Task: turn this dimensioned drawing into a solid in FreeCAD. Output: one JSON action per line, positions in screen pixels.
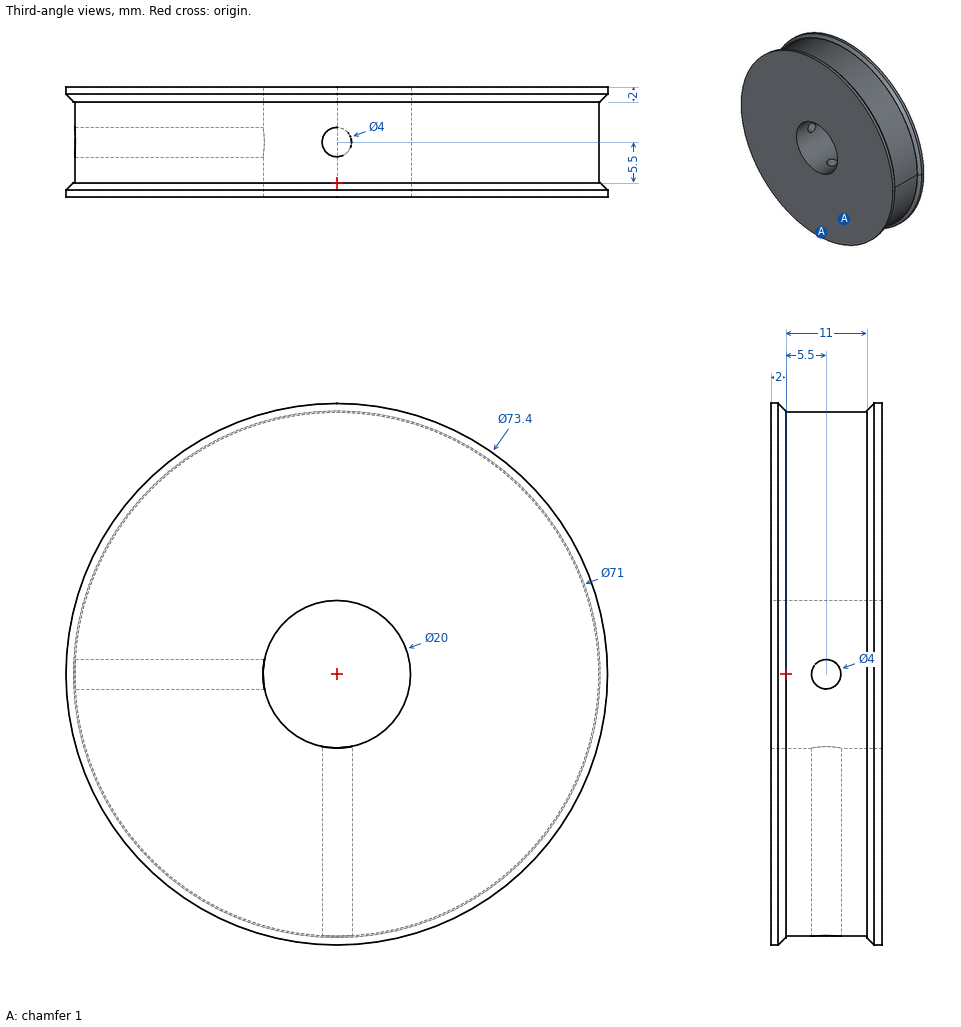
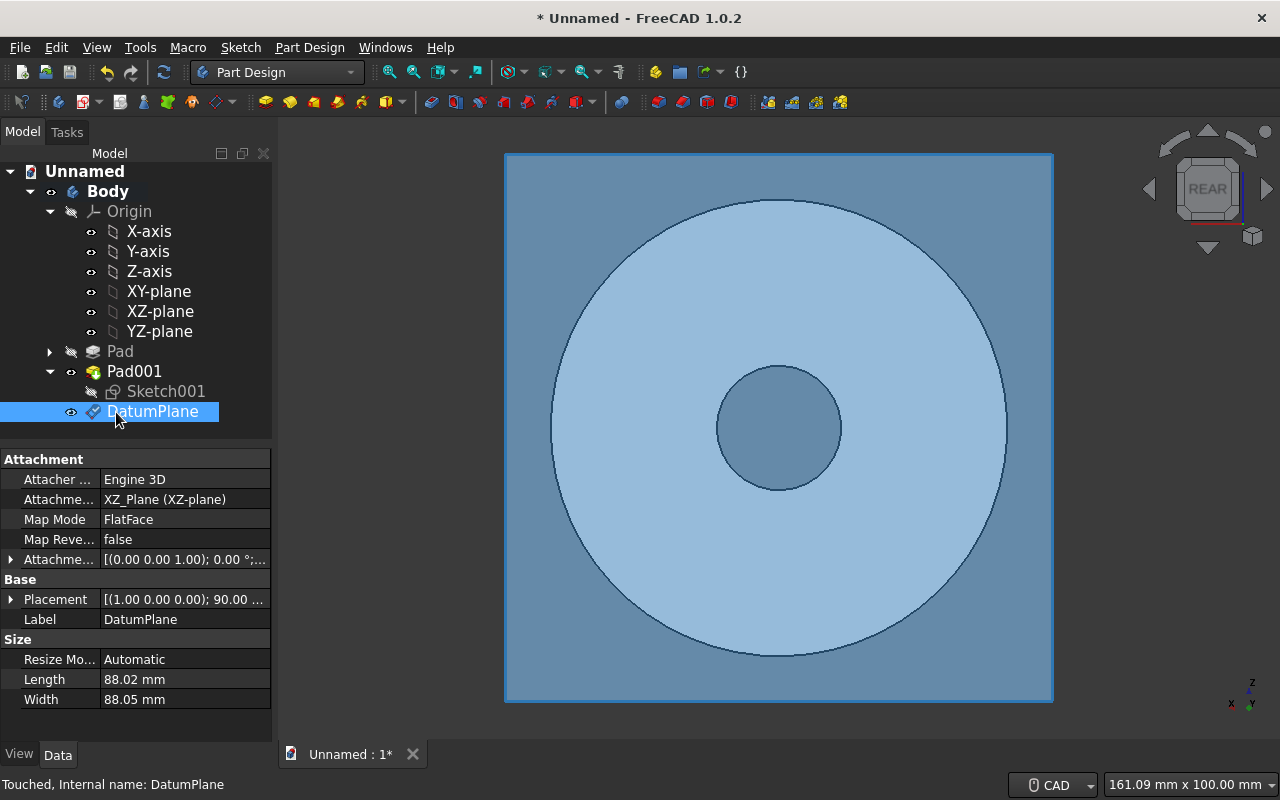
{"action": "left_click", "coordinate": [84, 102]}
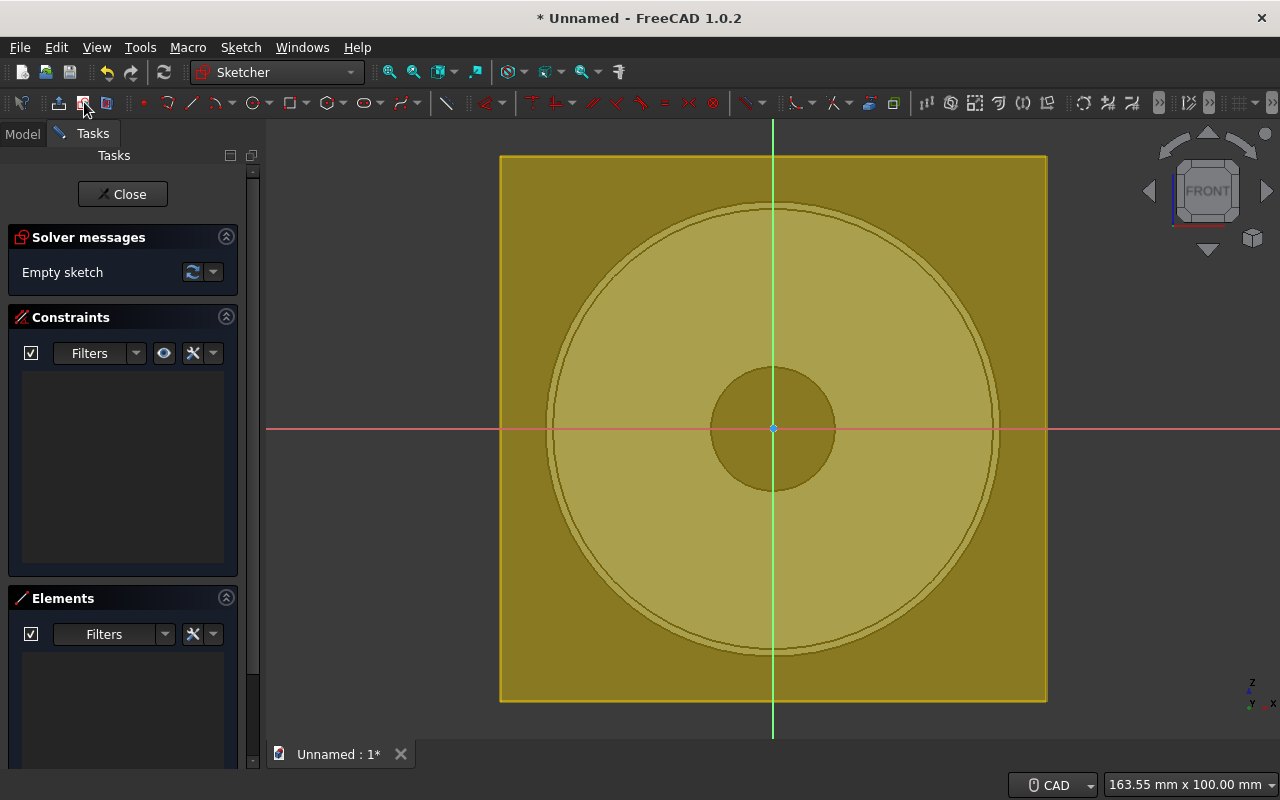
{"action": "left_click", "coordinate": [254, 104]}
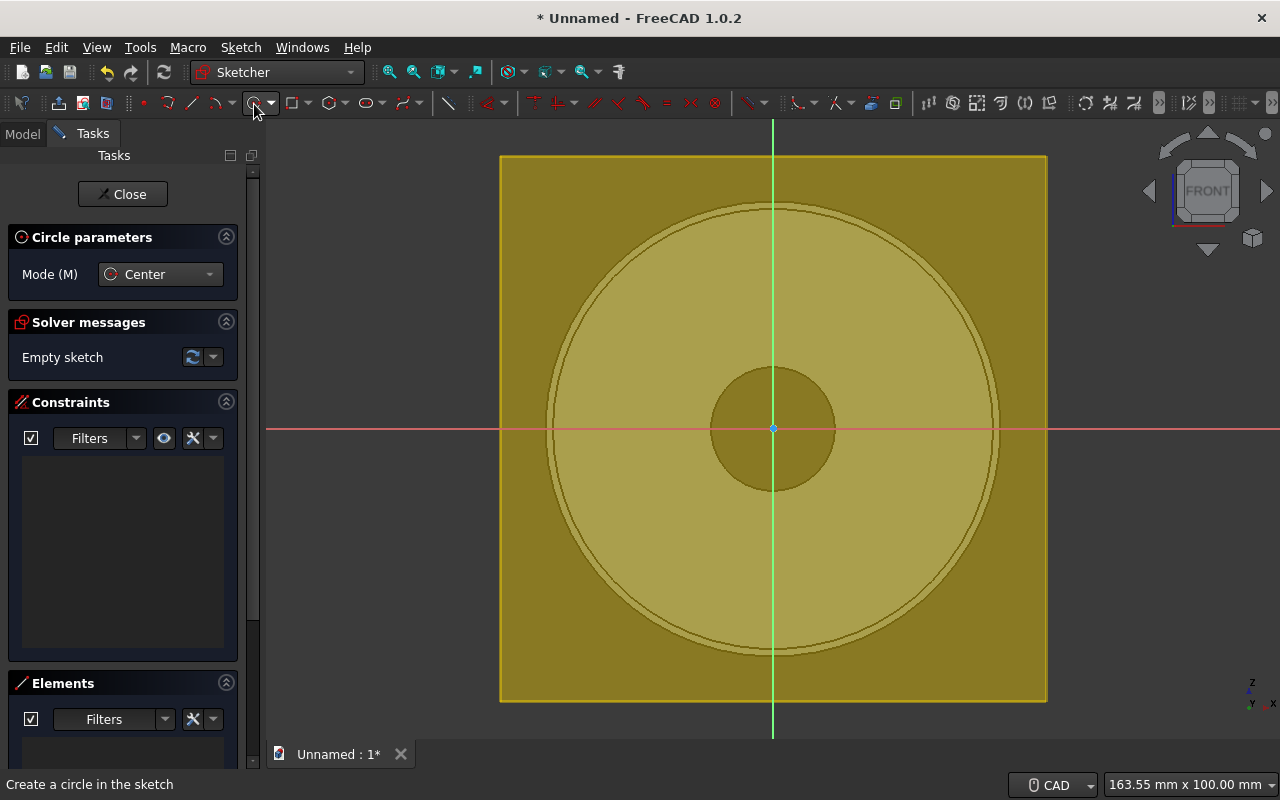
{"action": "left_click", "coordinate": [773, 429]}
{"action": "left_click", "coordinate": [934, 268]}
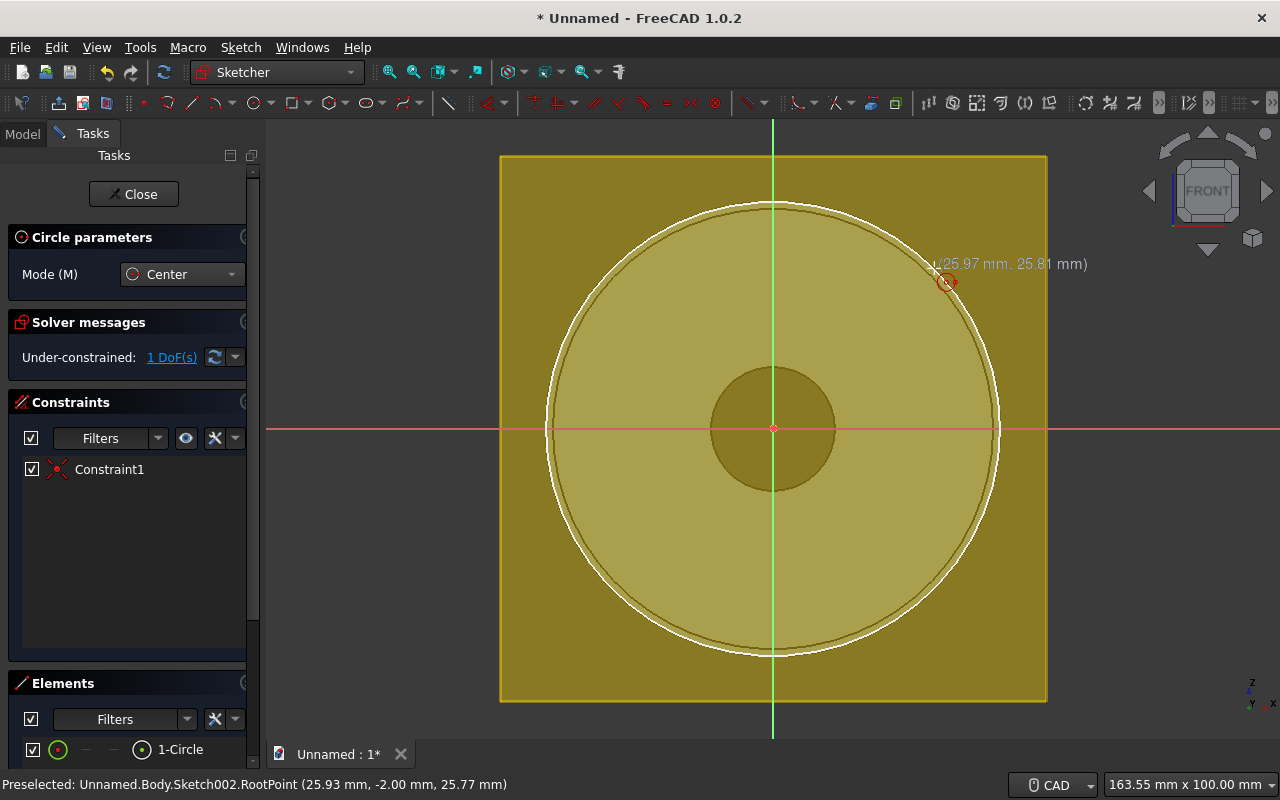
{"action": "left_click", "coordinate": [773, 429]}
{"action": "left_click", "coordinate": [817, 385]}
{"action": "key", "text": "Escape"}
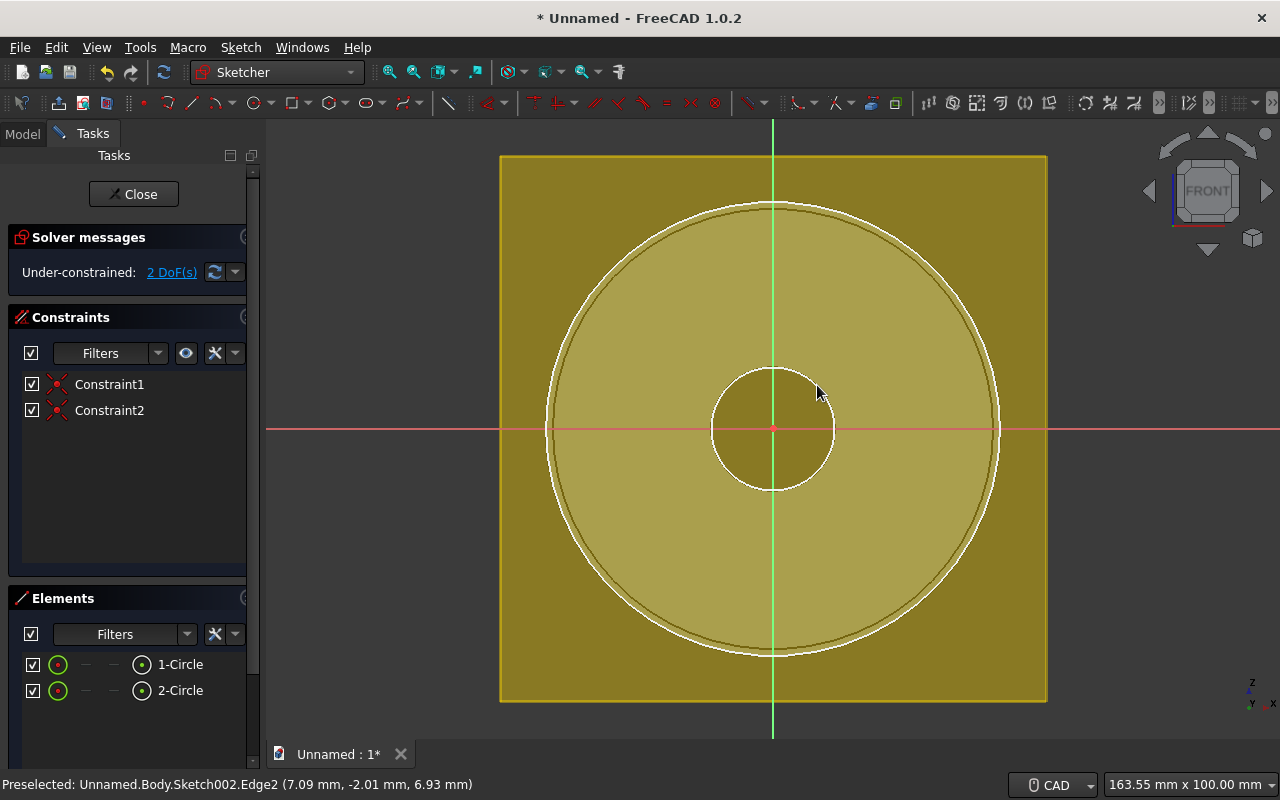
{"action": "left_click", "coordinate": [488, 104]}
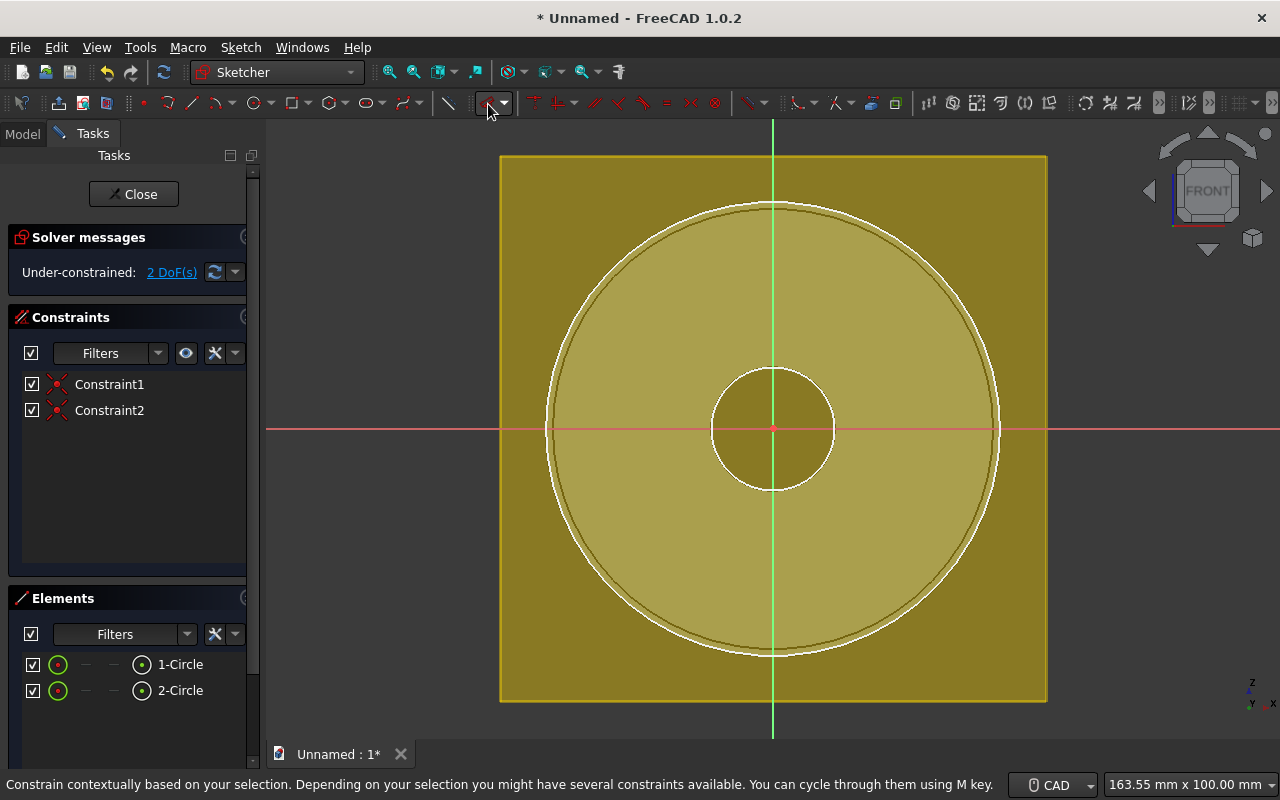
{"action": "left_click", "coordinate": [933, 268]}
{"action": "left_click", "coordinate": [956, 245]}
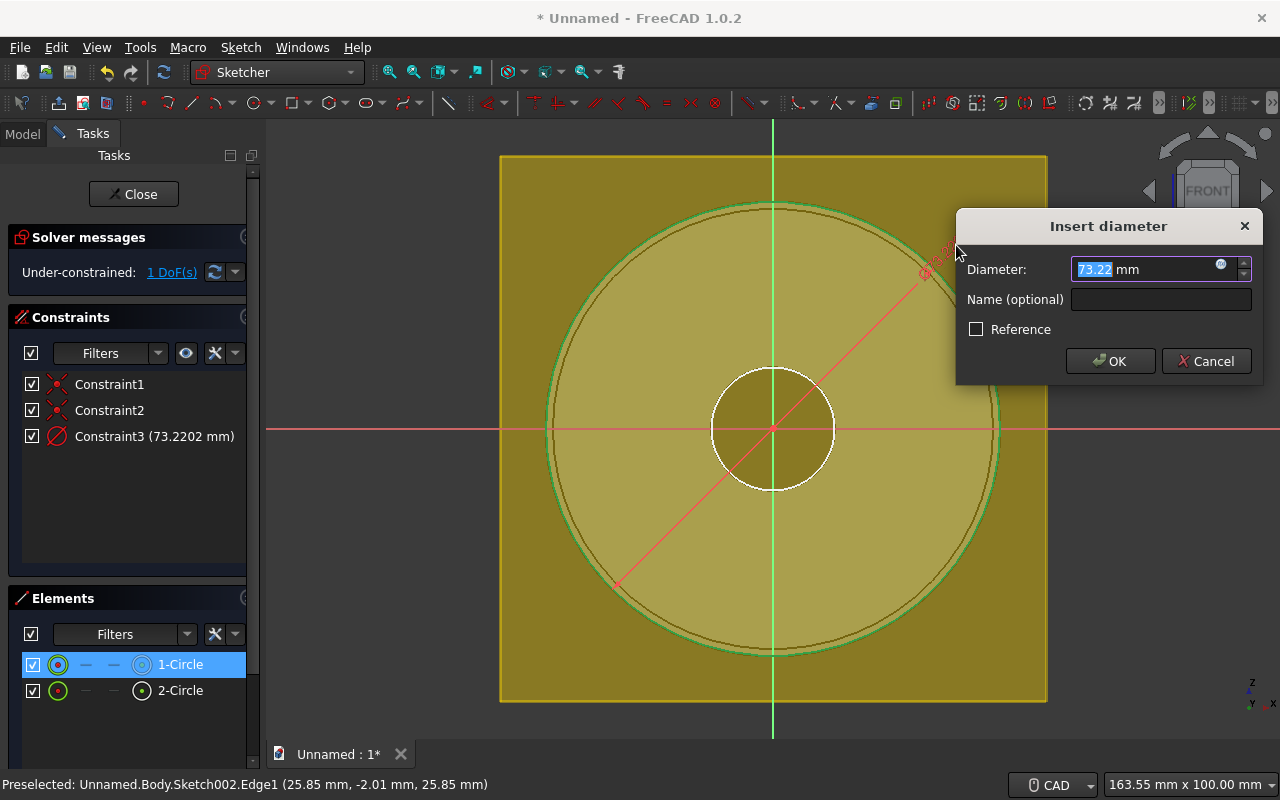
{"action": "type", "text": "73.4"}
{"action": "key", "text": "Return"}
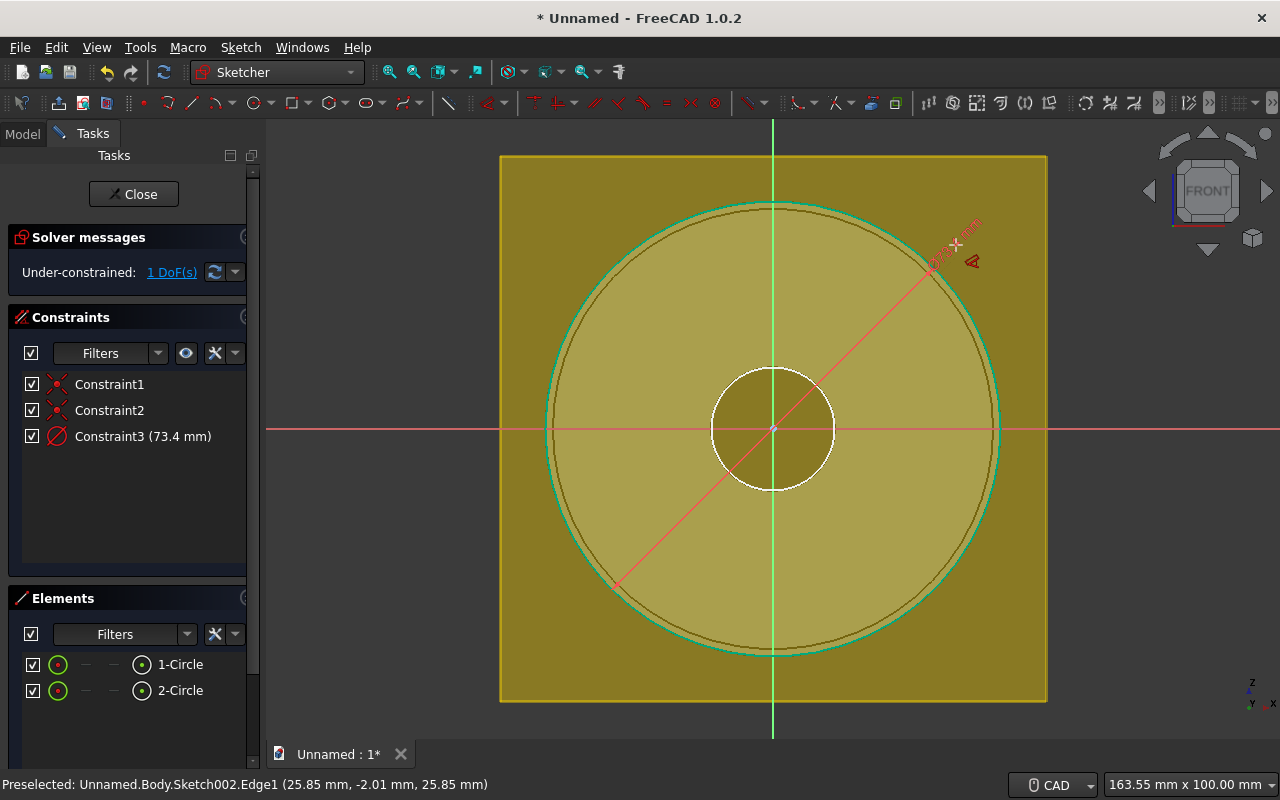
{"action": "left_click", "coordinate": [816, 385]}
{"action": "left_click", "coordinate": [838, 362]}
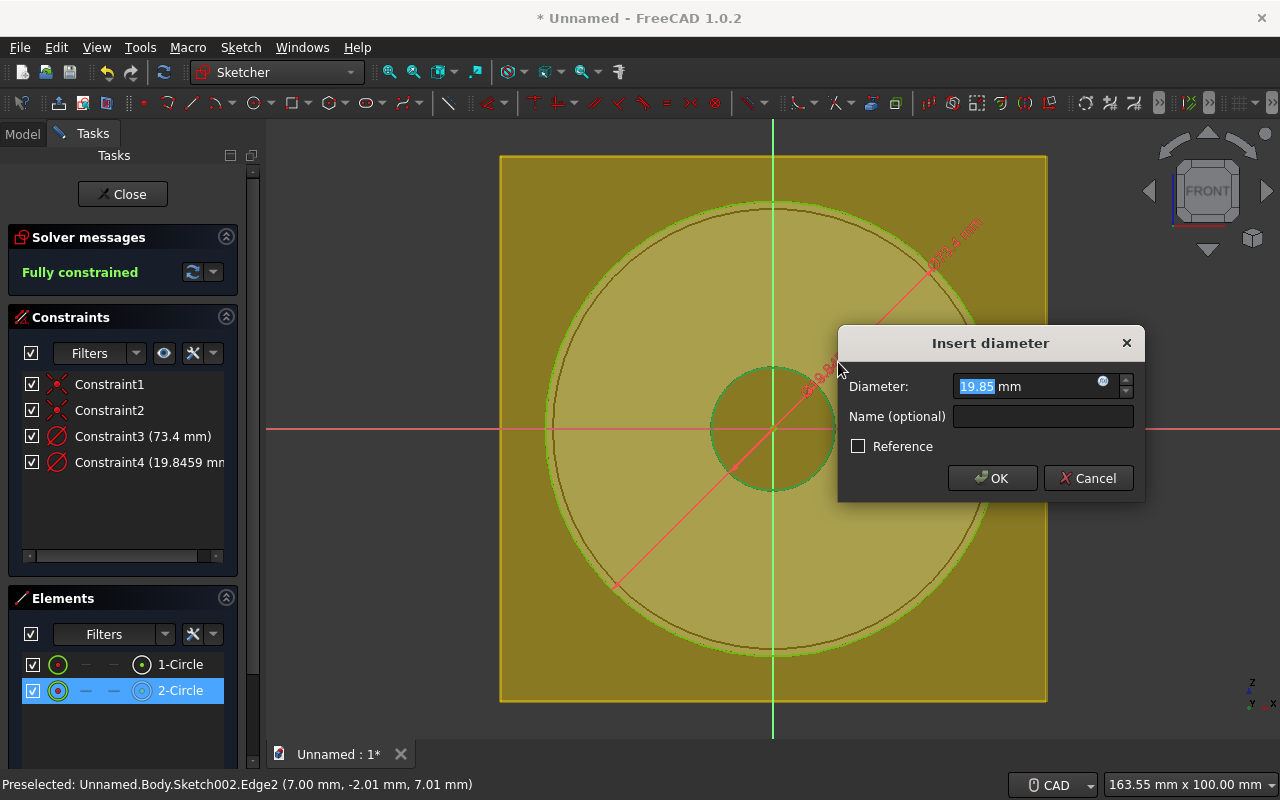
{"action": "type", "text": "20"}
{"action": "key", "text": "Return"}
{"action": "key", "text": "Escape"}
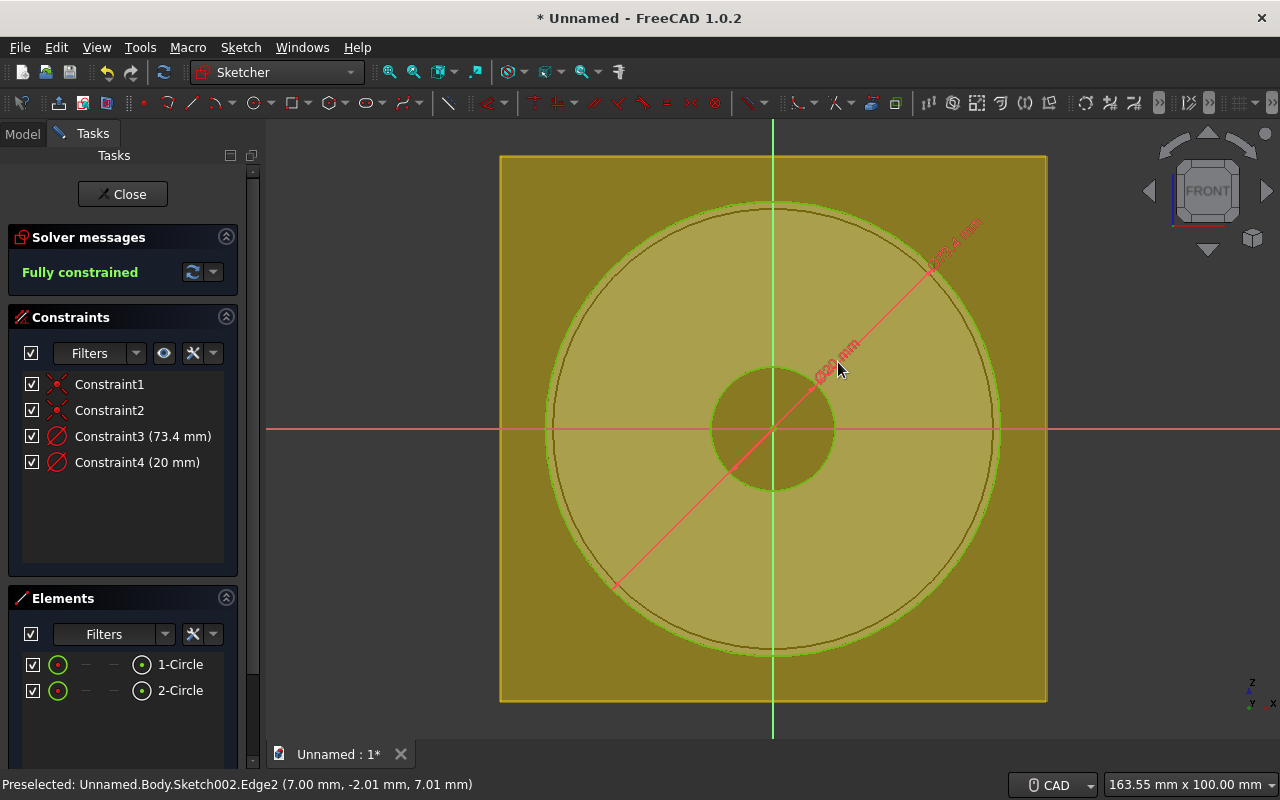
{"action": "left_click", "coordinate": [123, 194]}